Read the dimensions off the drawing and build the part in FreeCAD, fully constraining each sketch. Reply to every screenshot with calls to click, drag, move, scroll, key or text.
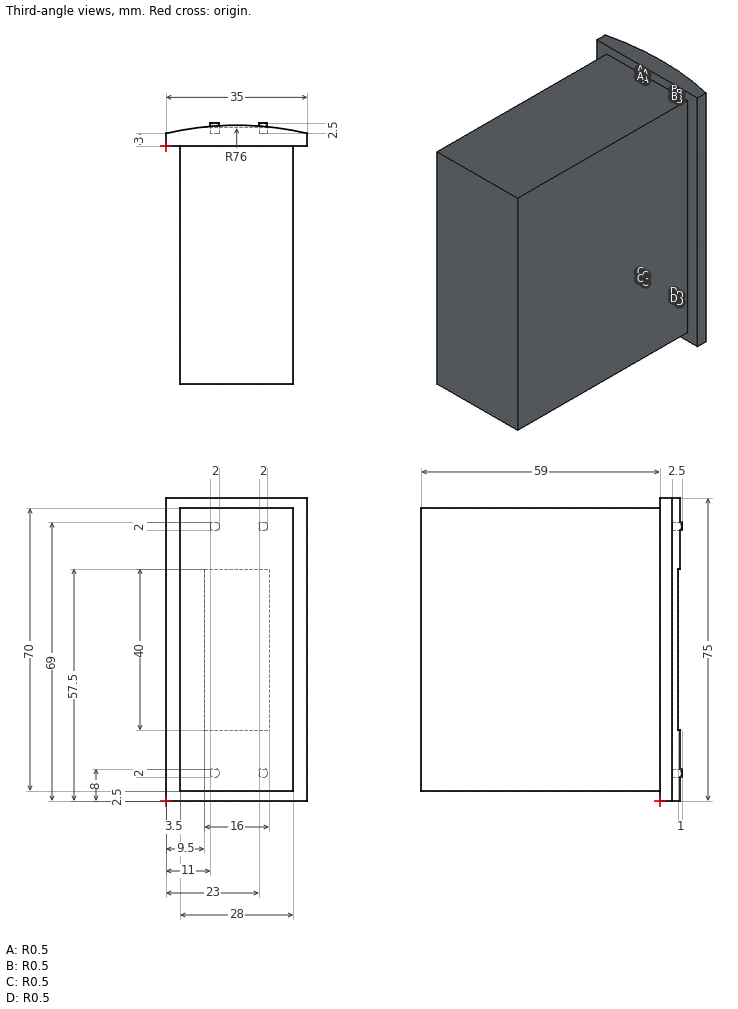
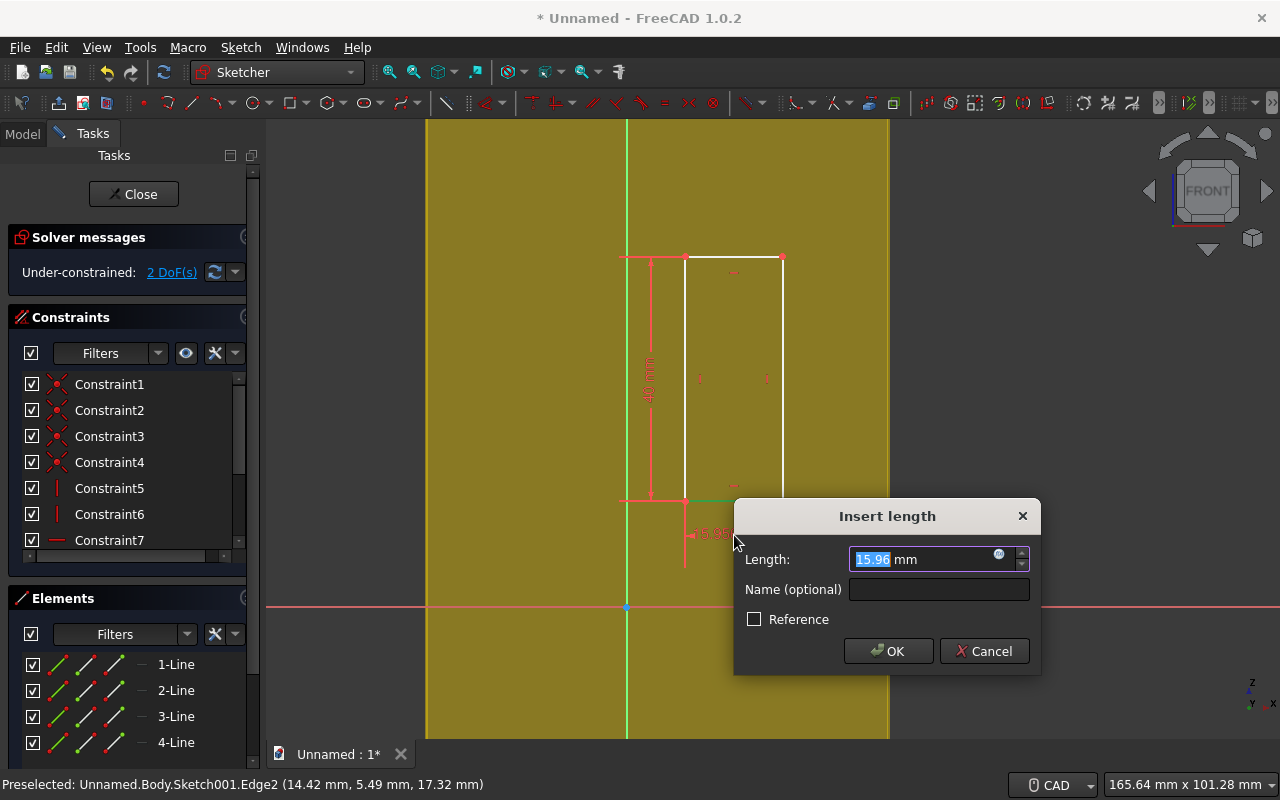
text(16)
key(Return)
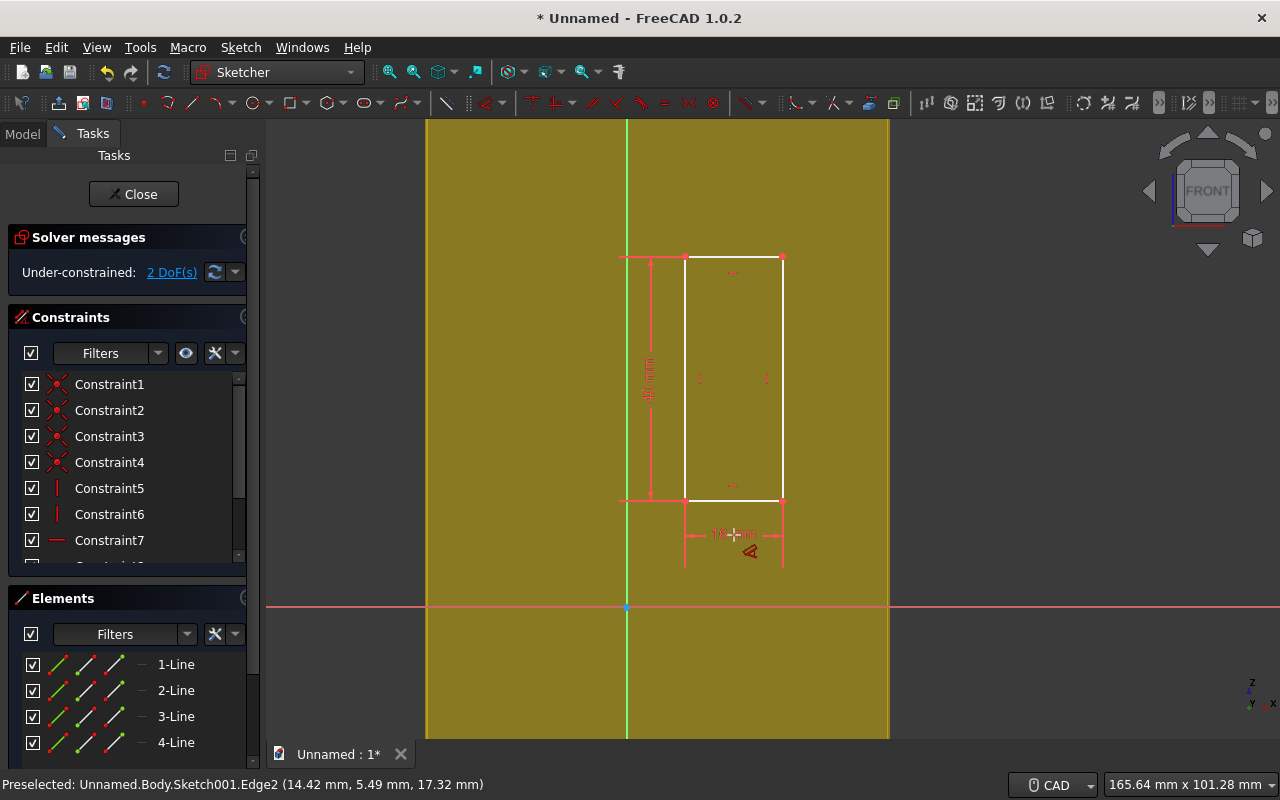
click(685, 257)
click(656, 641)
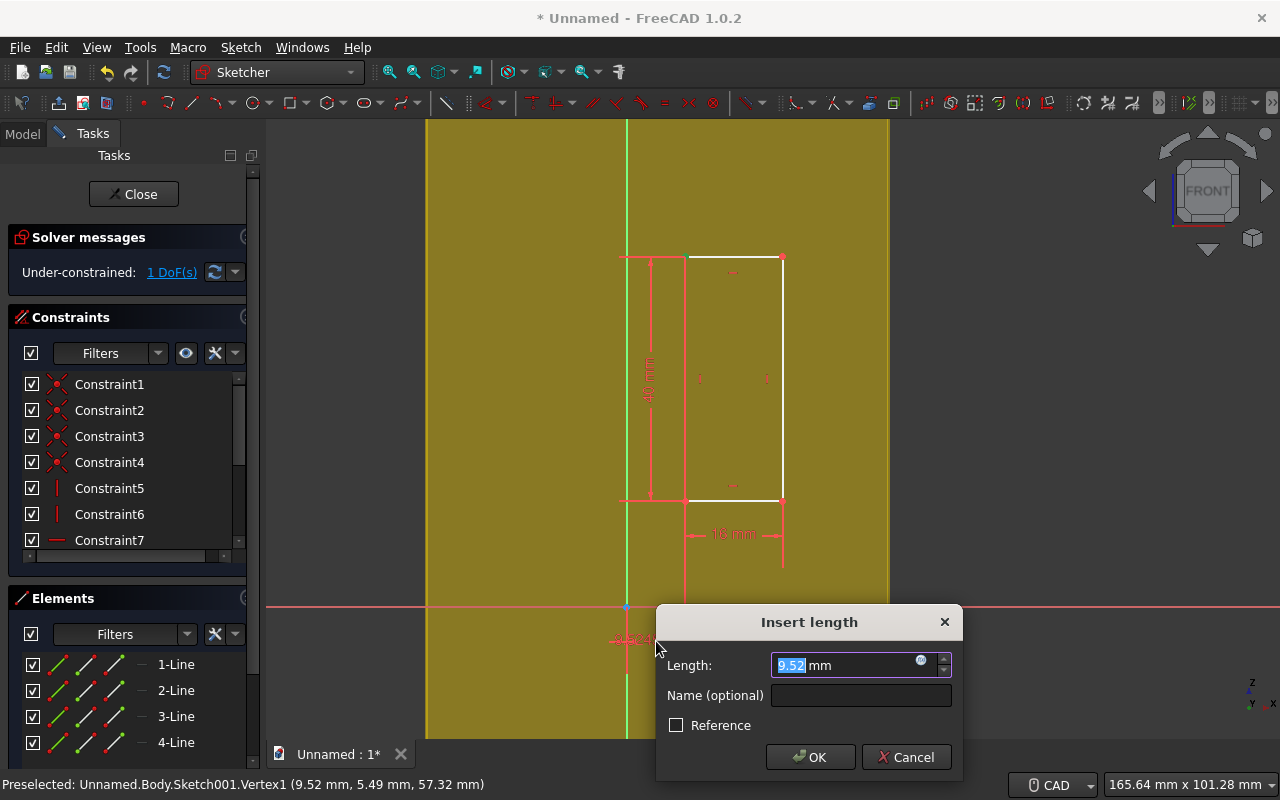
text(9.5)
key(Return)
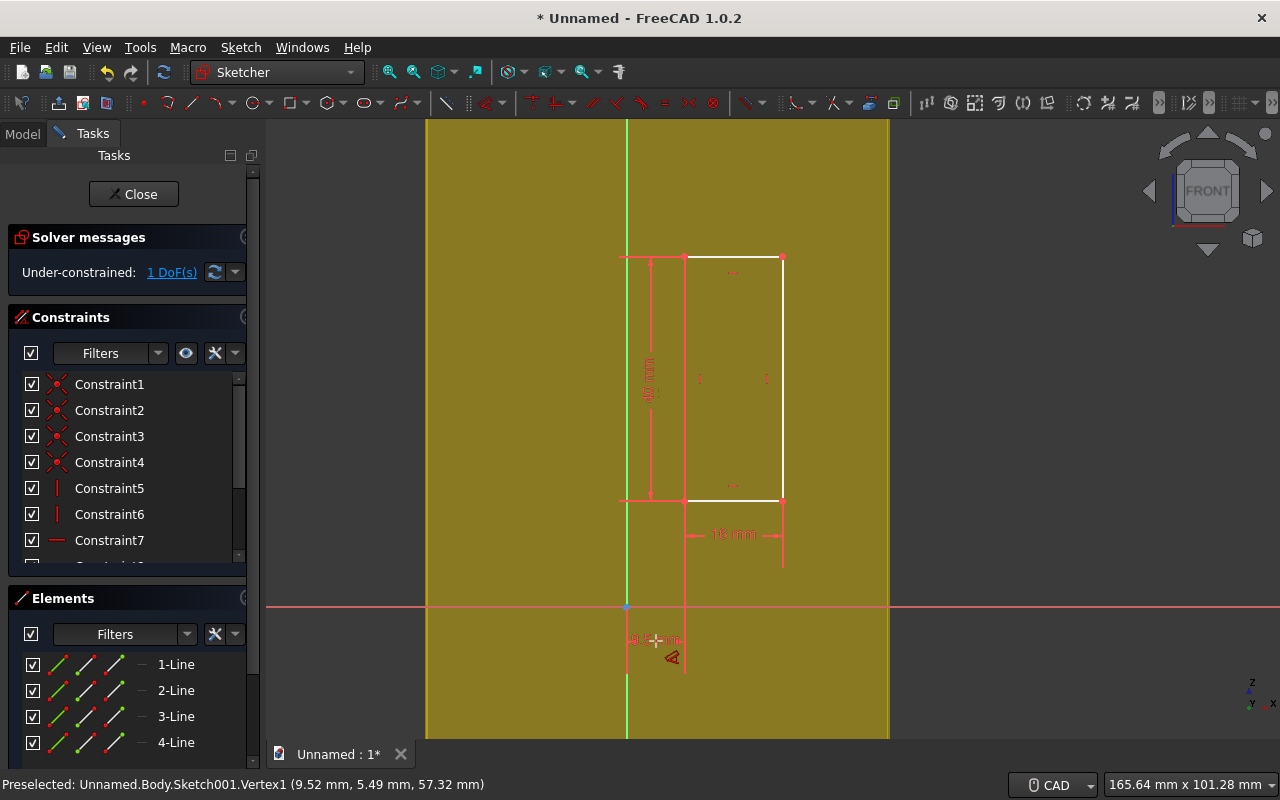
click(685, 257)
click(593, 432)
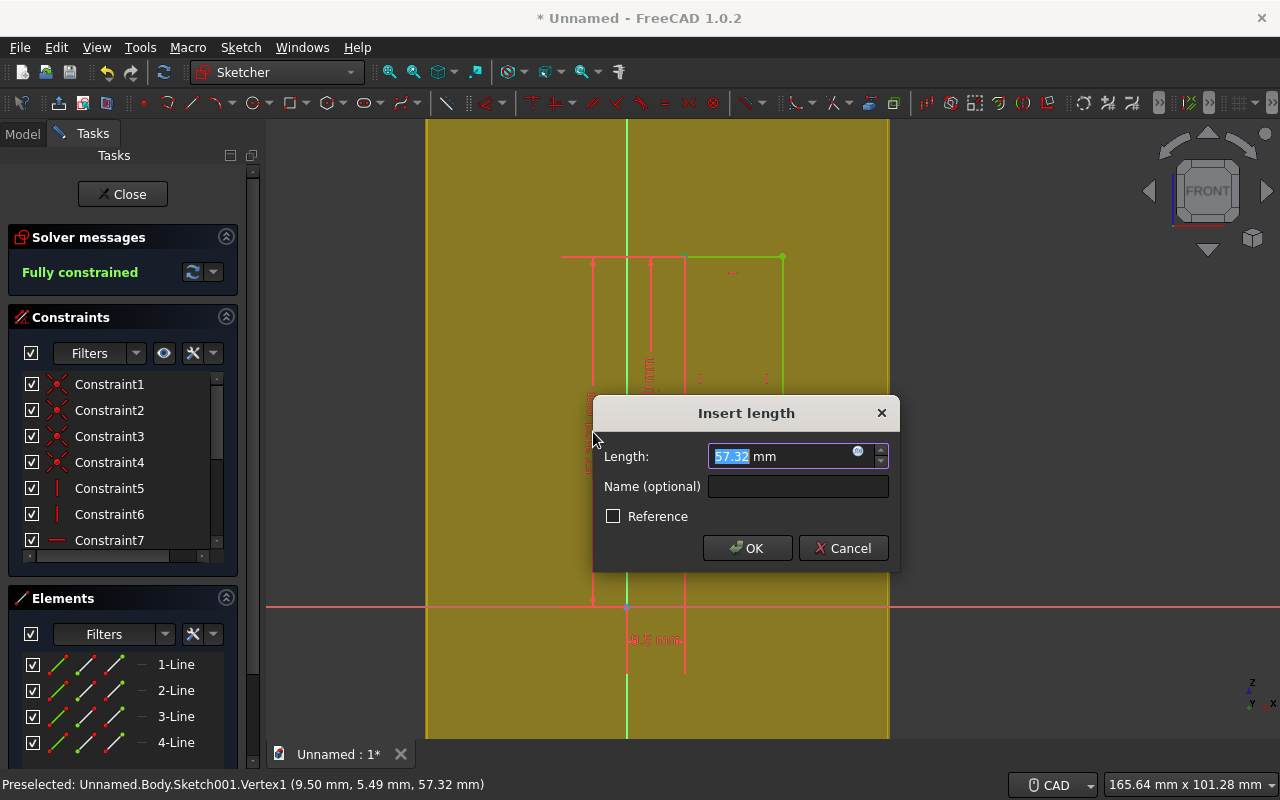
text(57.5)
key(Return)
key(Escape)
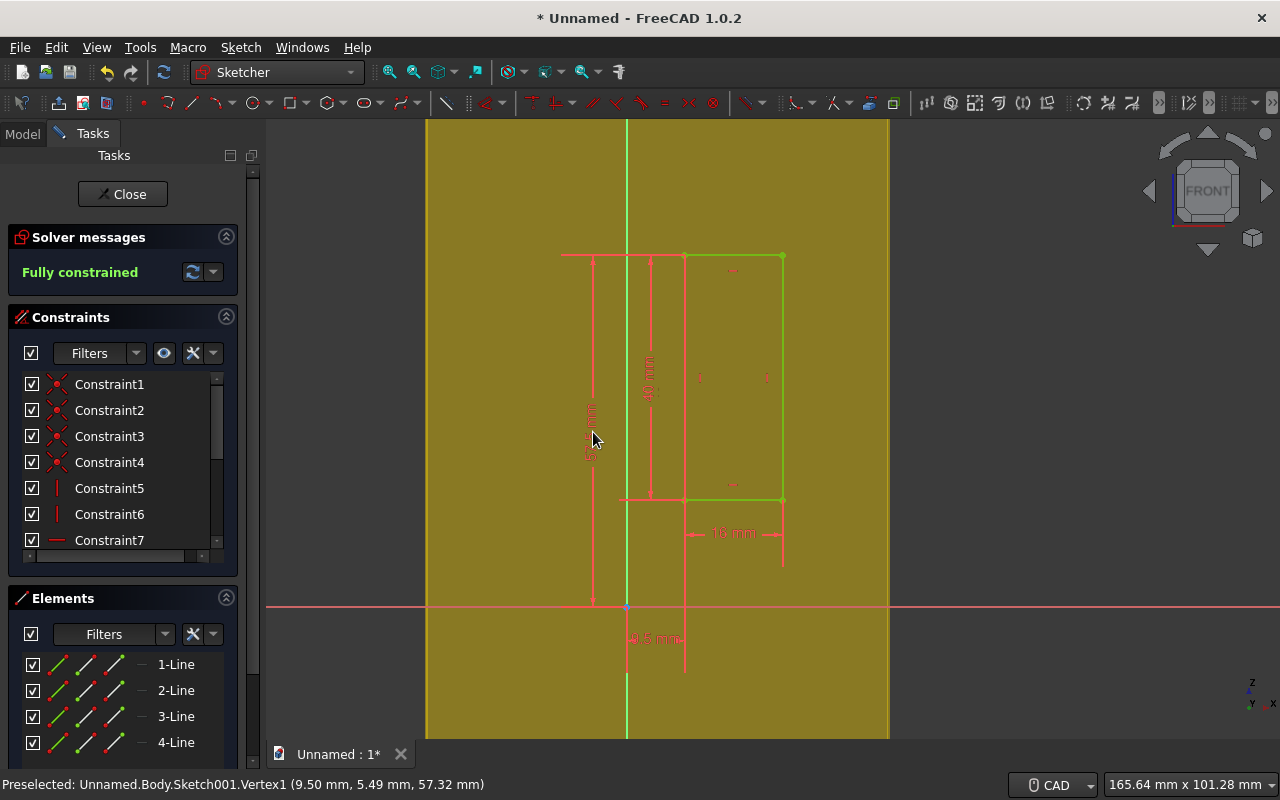
click(123, 194)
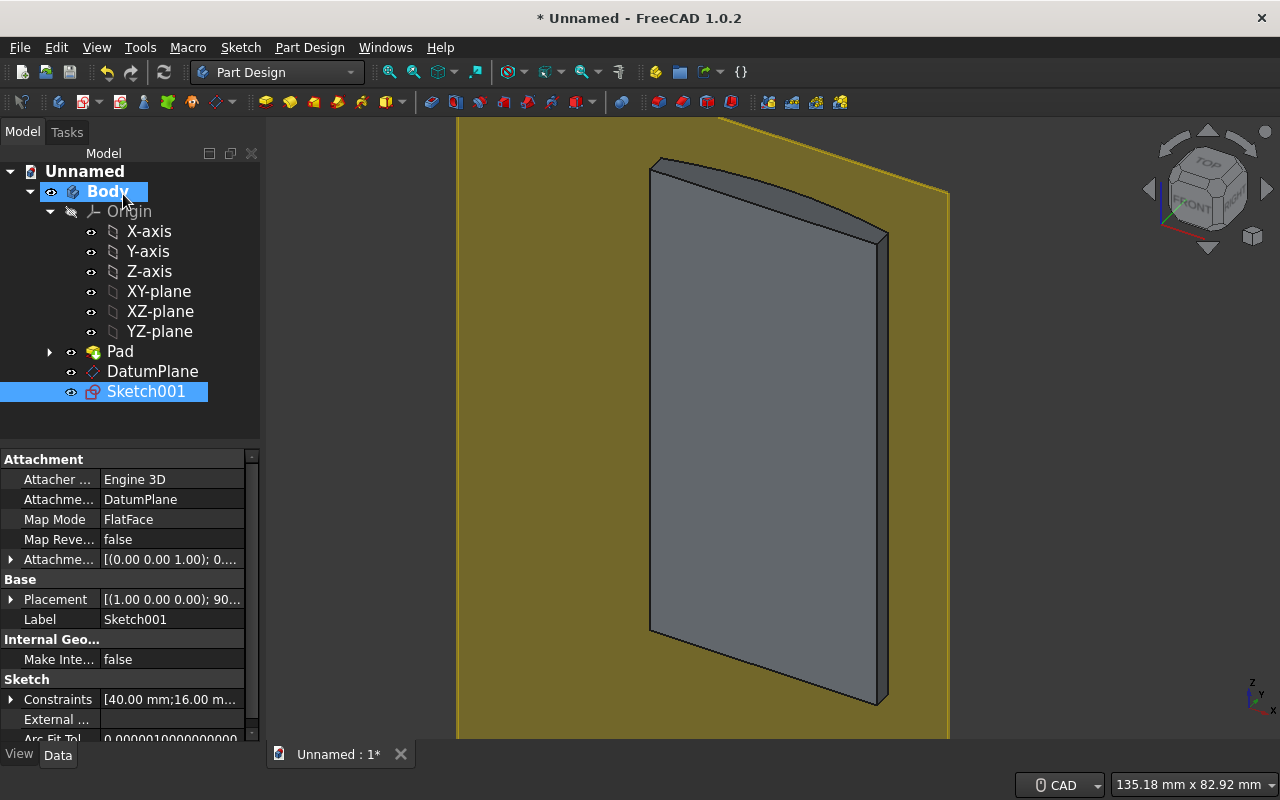
click(432, 102)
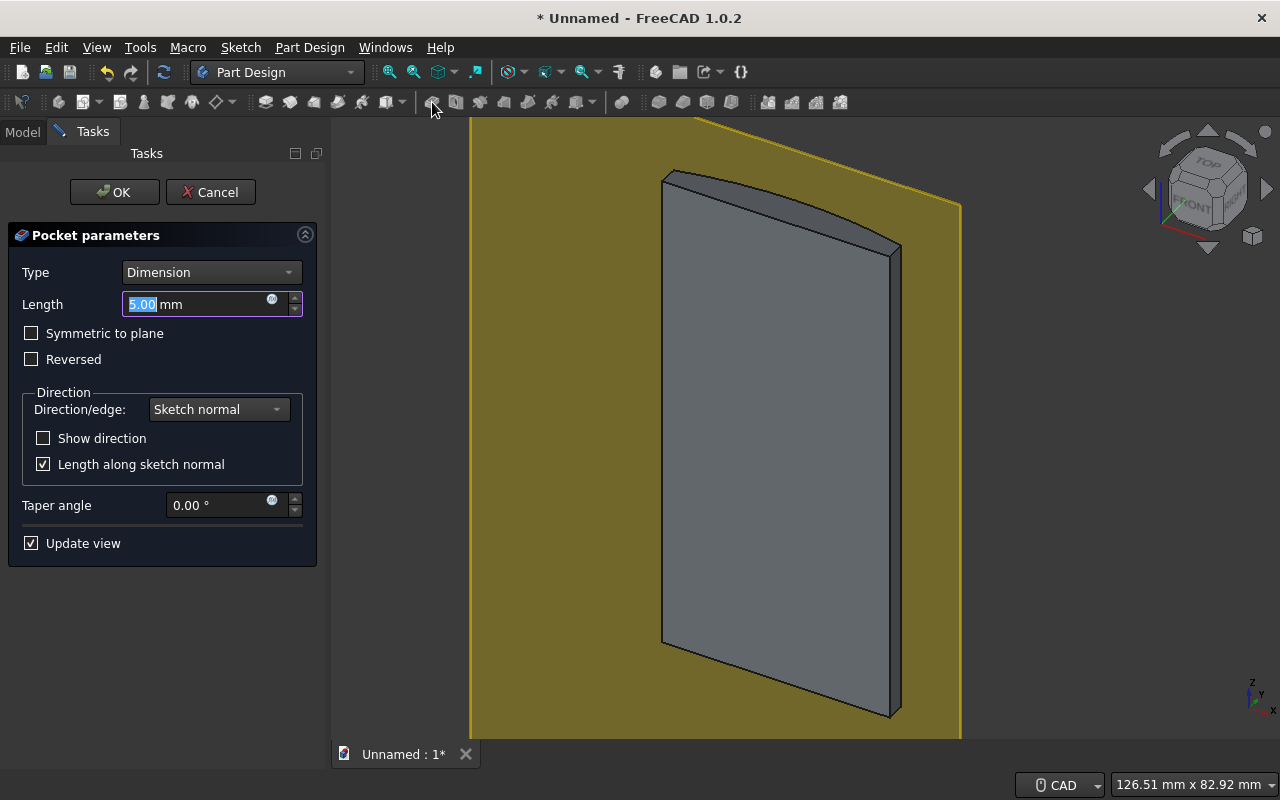
text(1)
key(Tab)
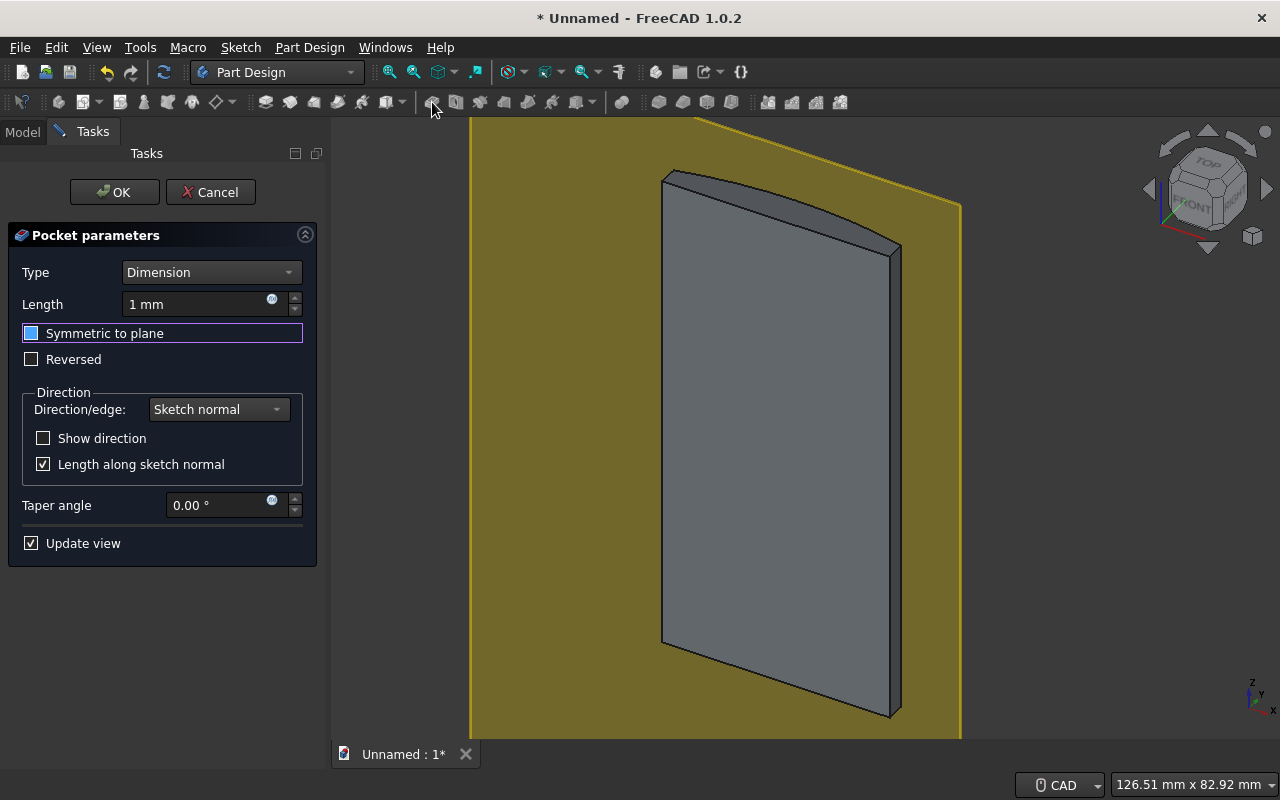
click(30, 359)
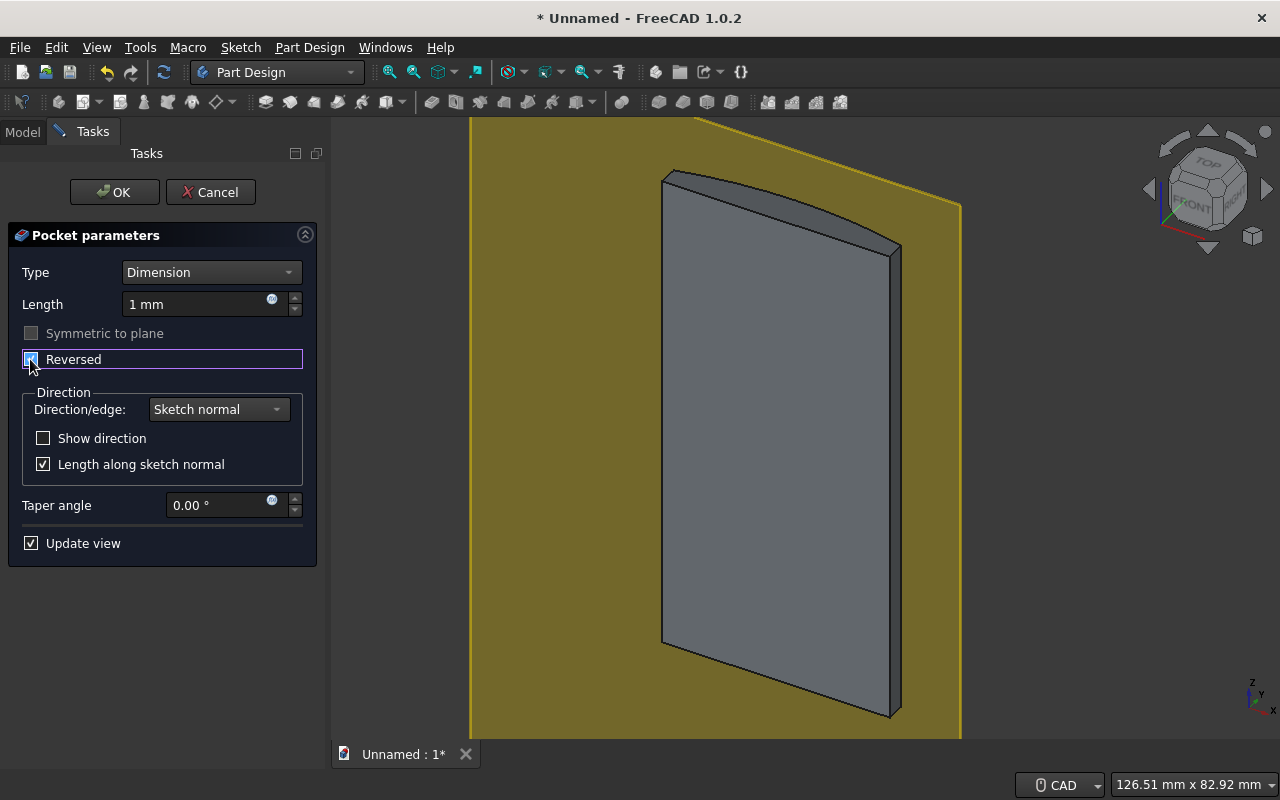
click(115, 192)